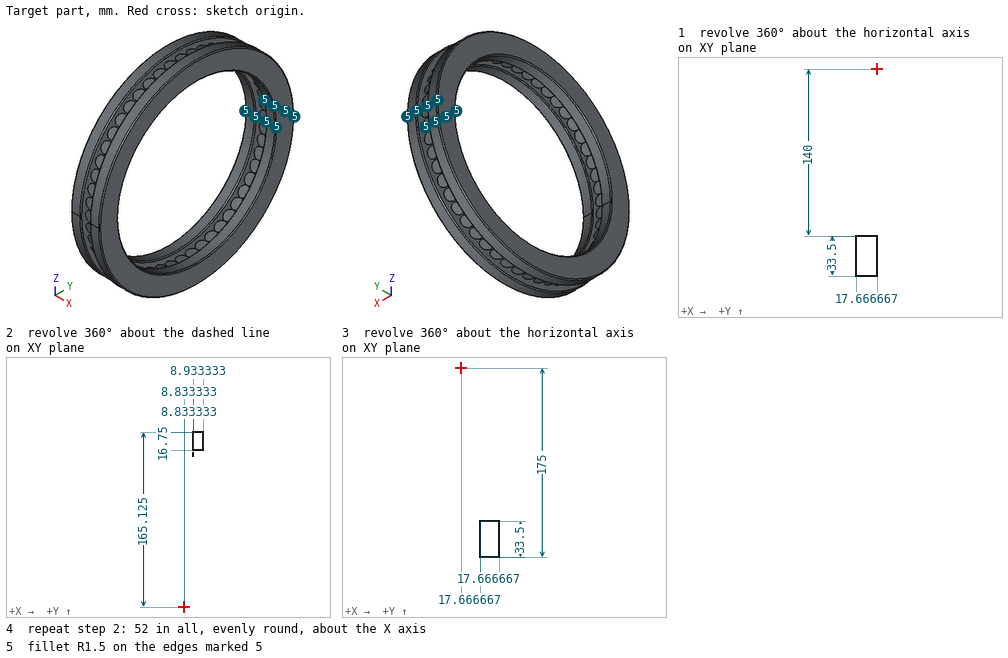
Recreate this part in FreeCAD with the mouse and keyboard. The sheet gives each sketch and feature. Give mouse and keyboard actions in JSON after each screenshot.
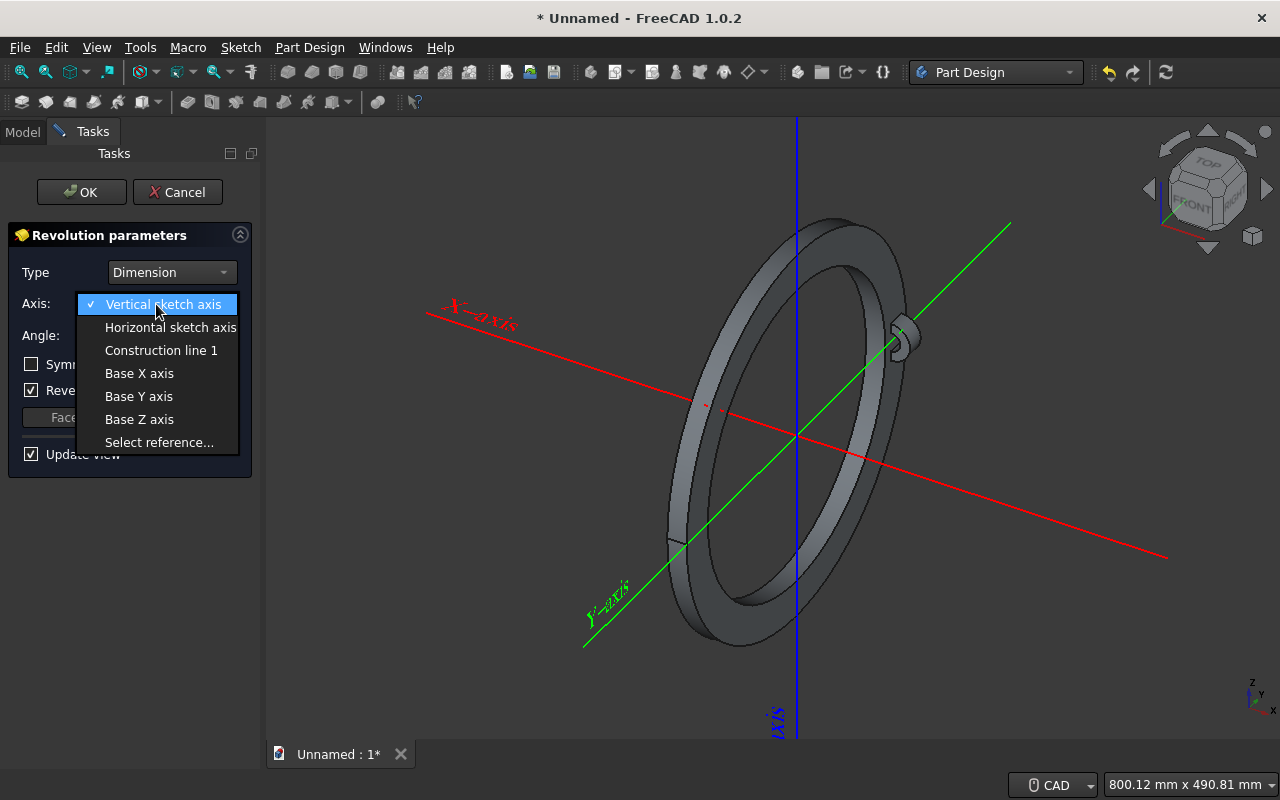
{"action": "left_click", "coordinate": [156, 350]}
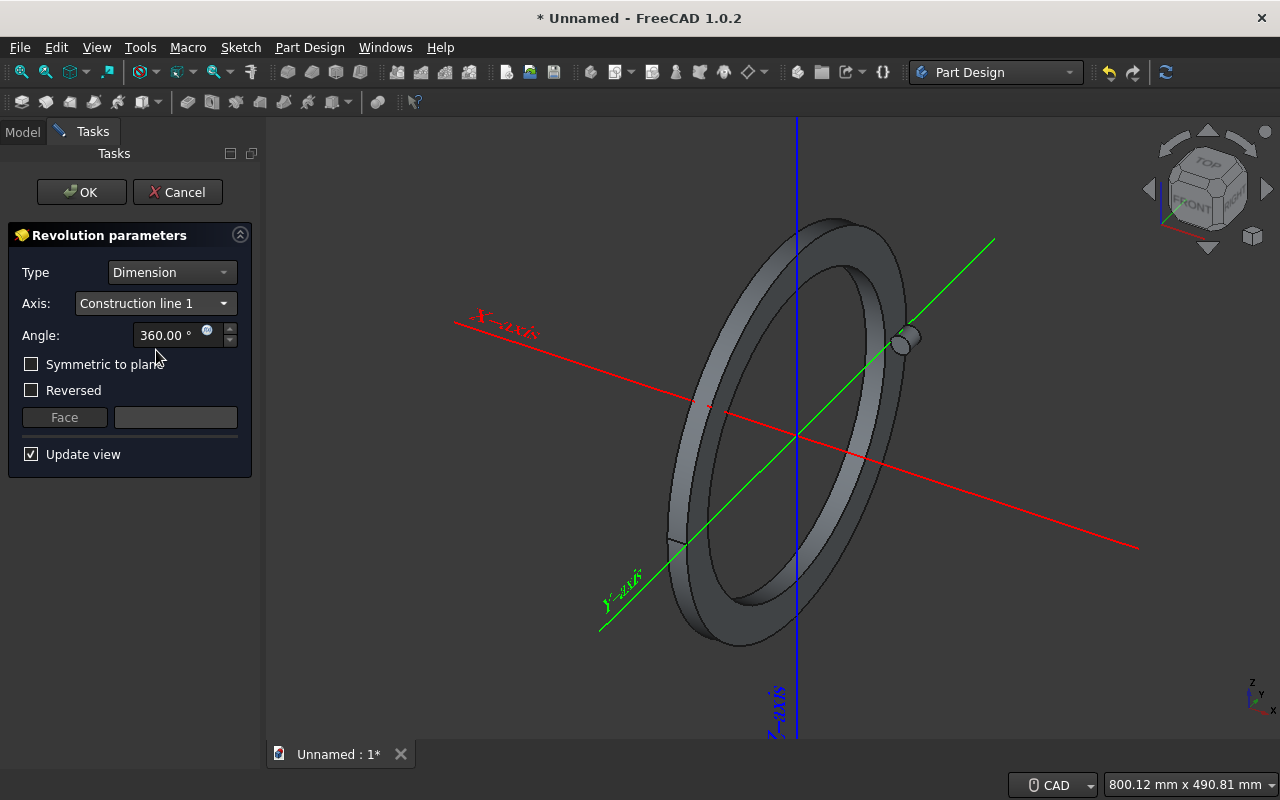
{"action": "left_click", "coordinate": [82, 192]}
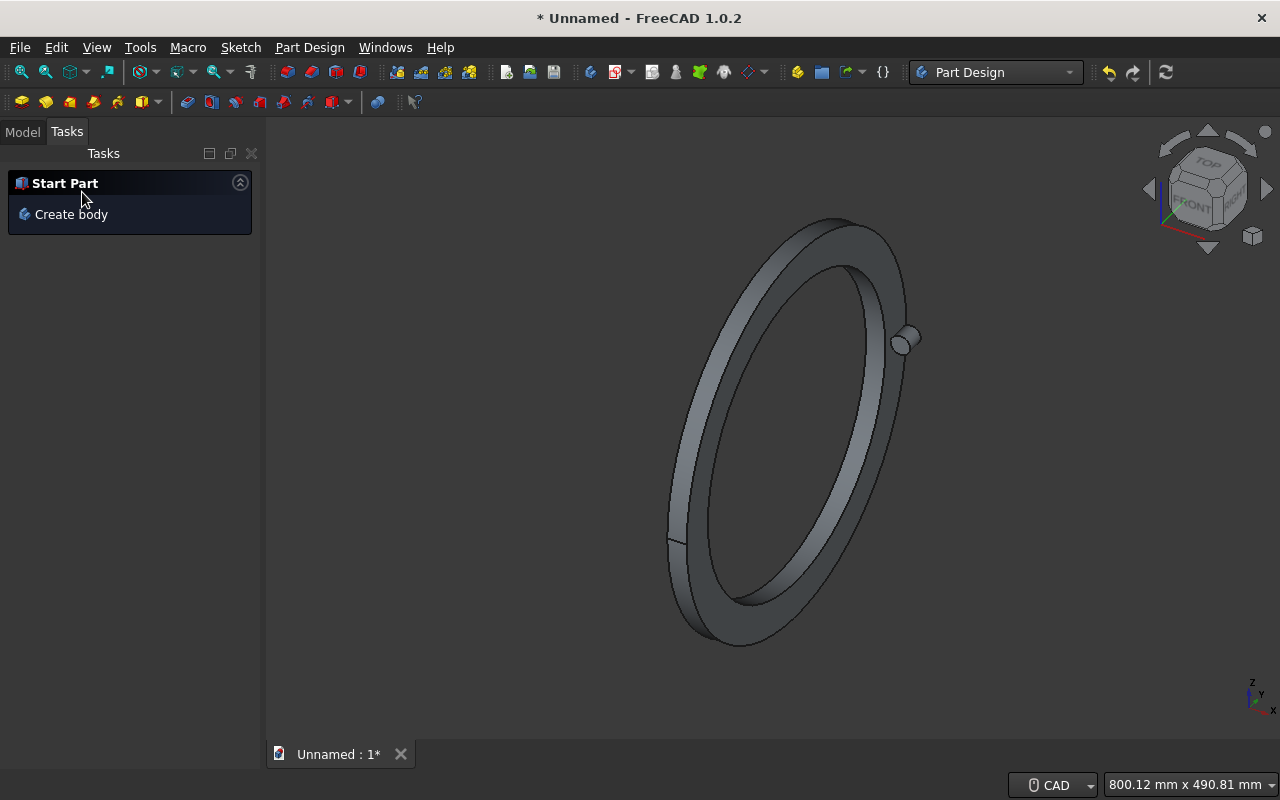
{"action": "left_click", "coordinate": [616, 72]}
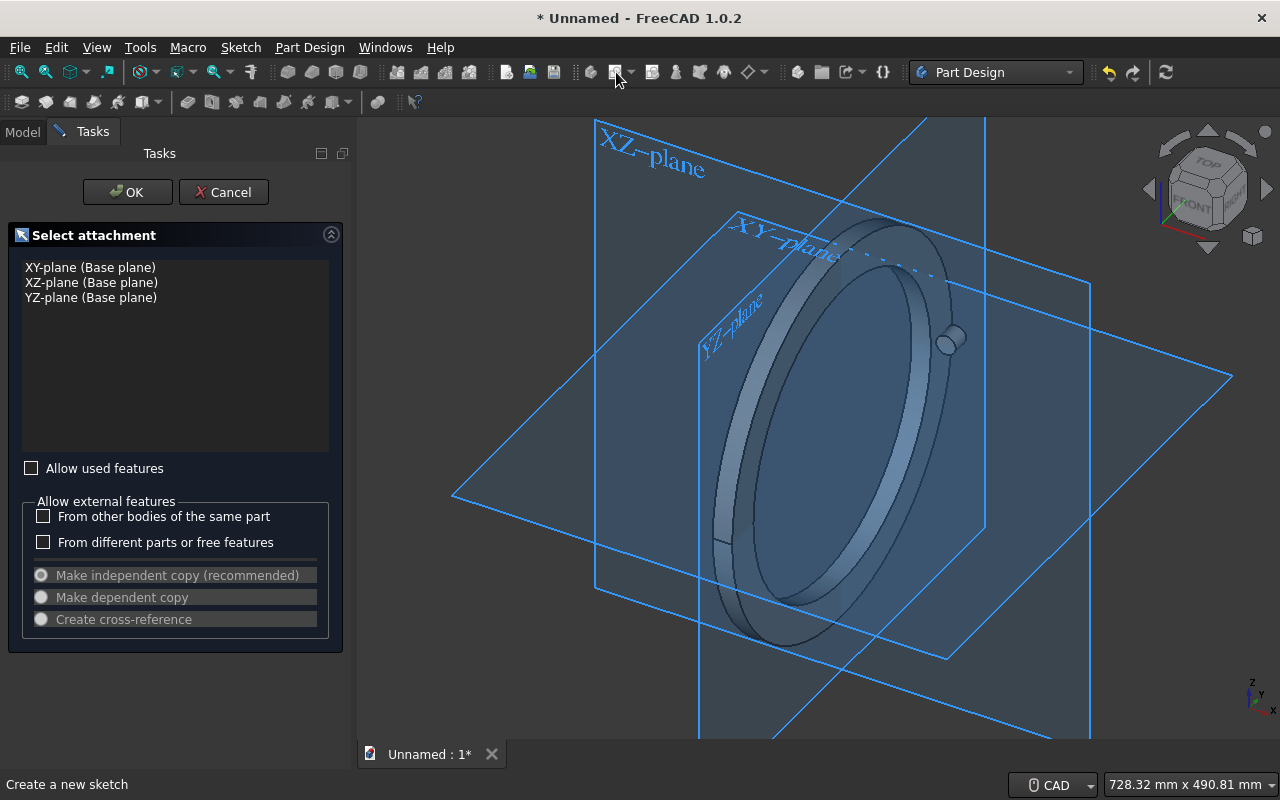
{"action": "left_click", "coordinate": [82, 268]}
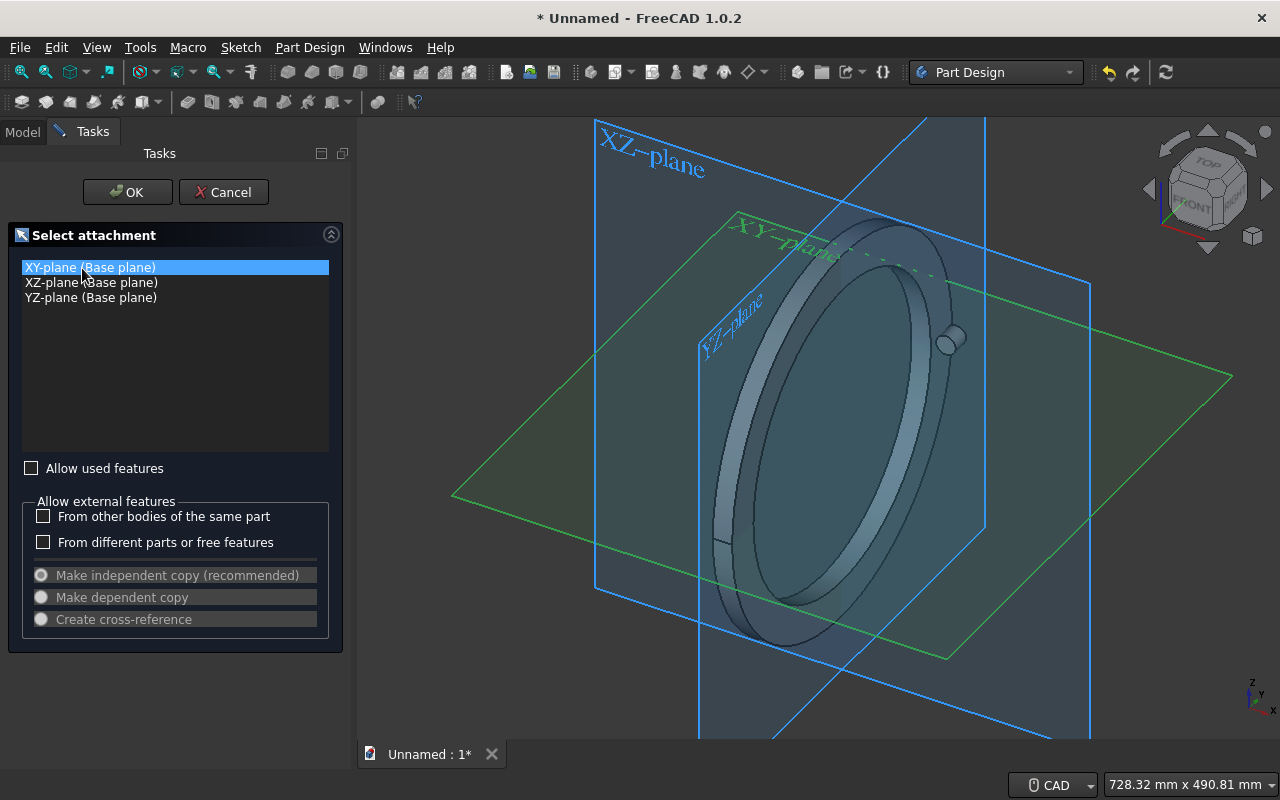
{"action": "left_click", "coordinate": [128, 192]}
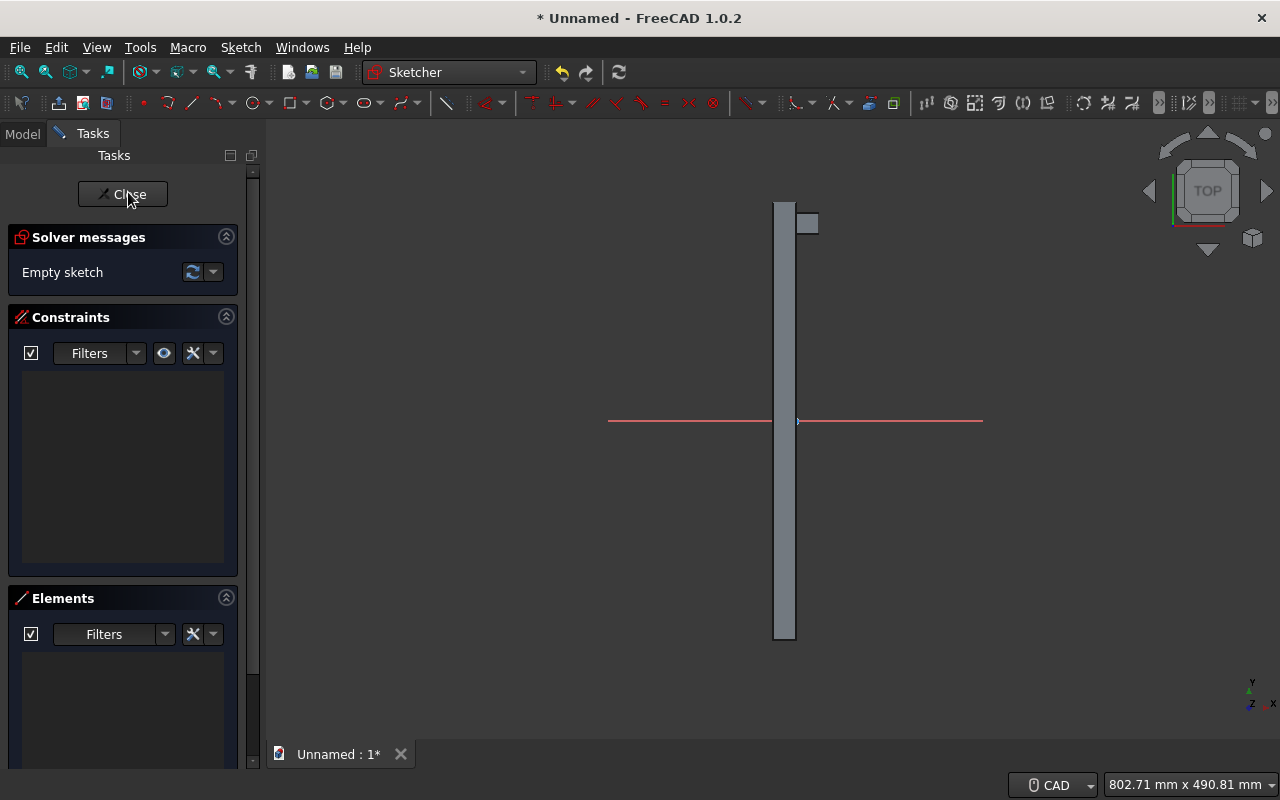
{"action": "left_click", "coordinate": [108, 104]}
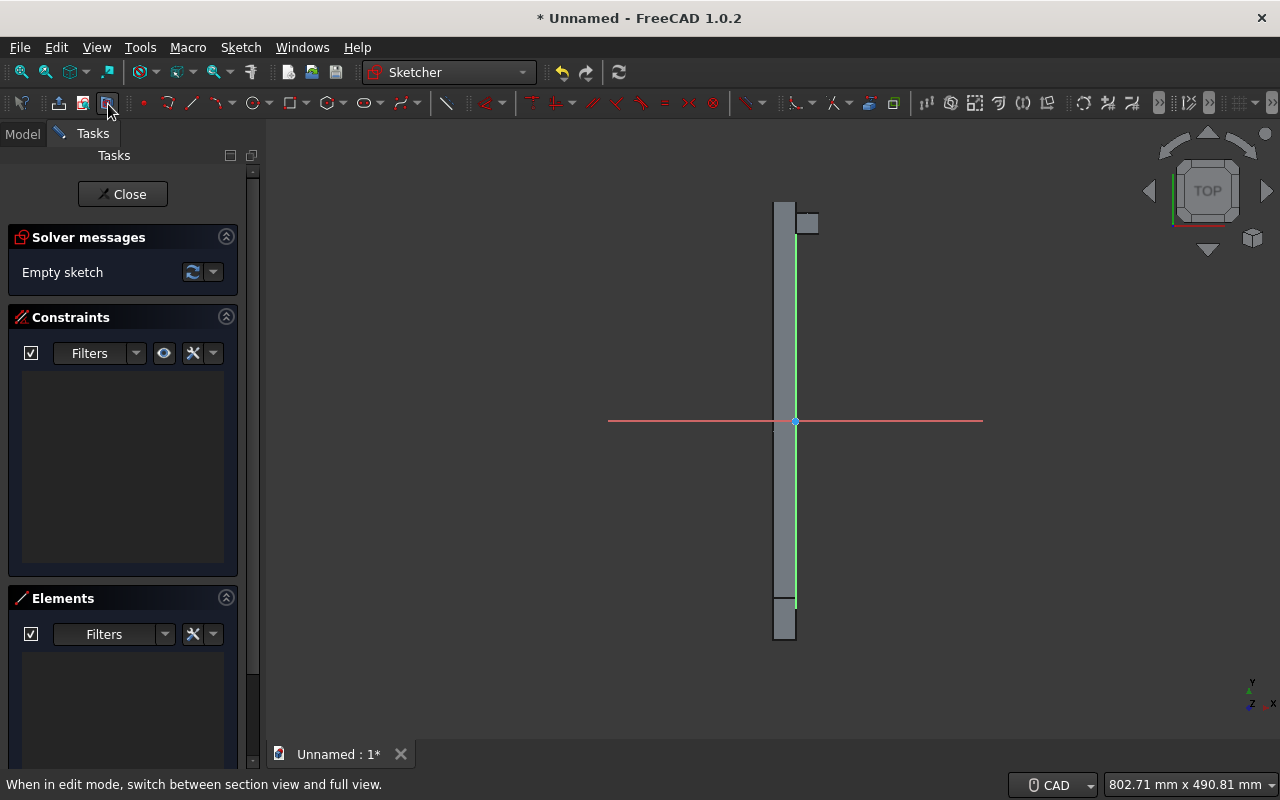
{"action": "scroll", "coordinate": [845, 645], "scroll_direction": "up", "scroll_amount": 11}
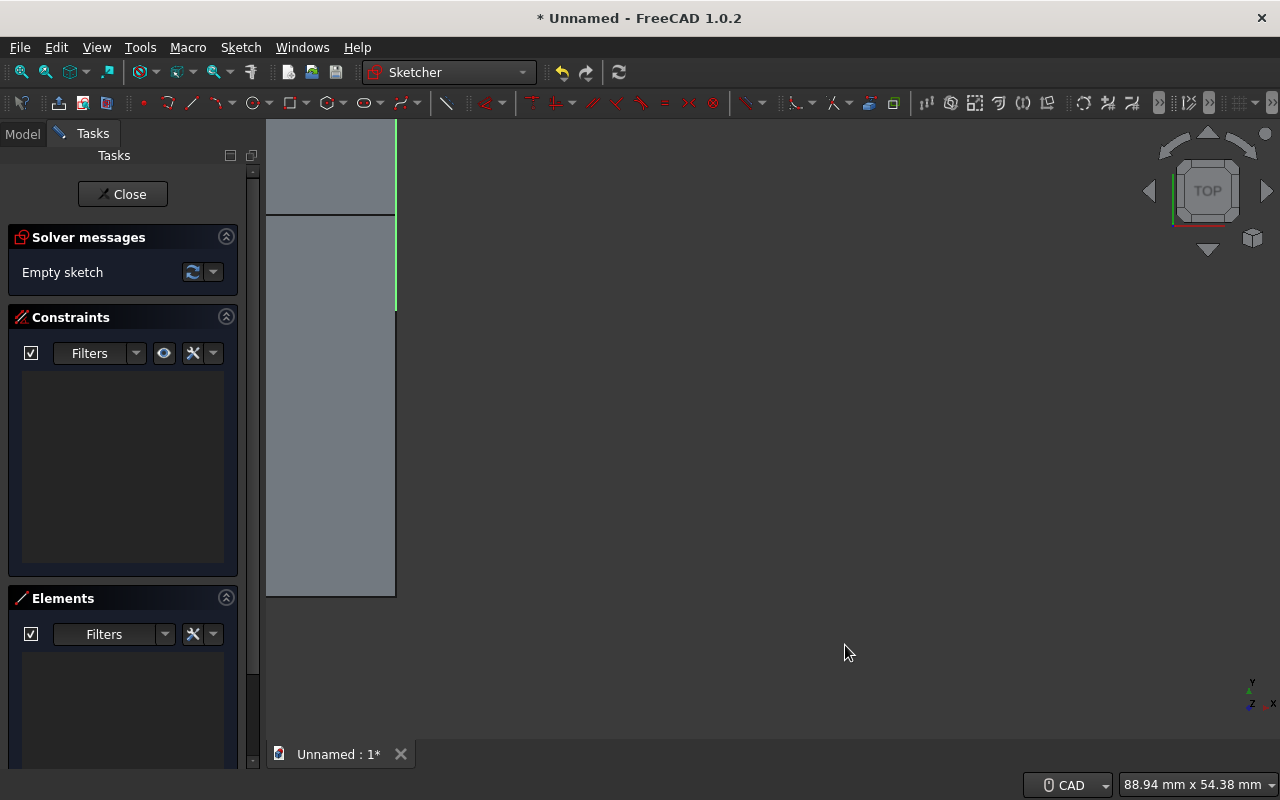
{"action": "left_click", "coordinate": [290, 104]}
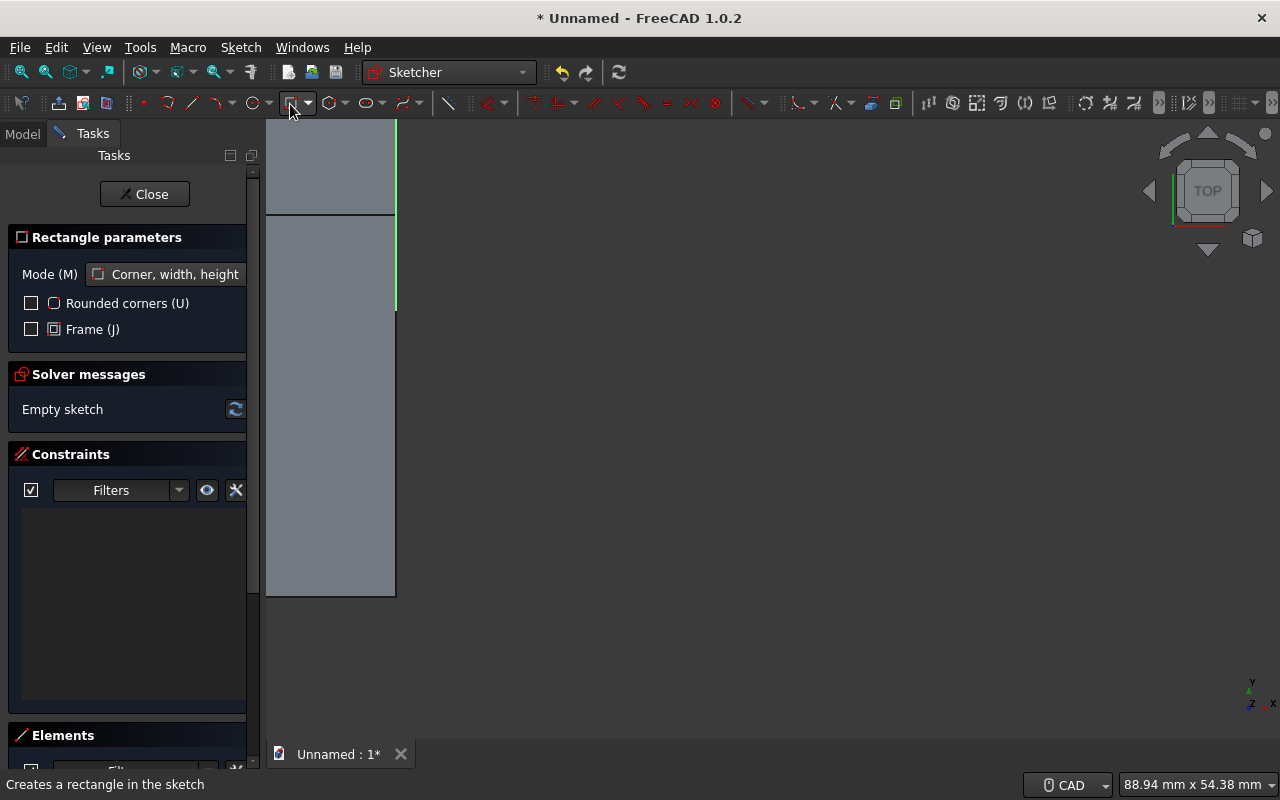
{"action": "left_click", "coordinate": [597, 232]}
{"action": "left_click", "coordinate": [799, 614]}
{"action": "key", "text": "Escape"}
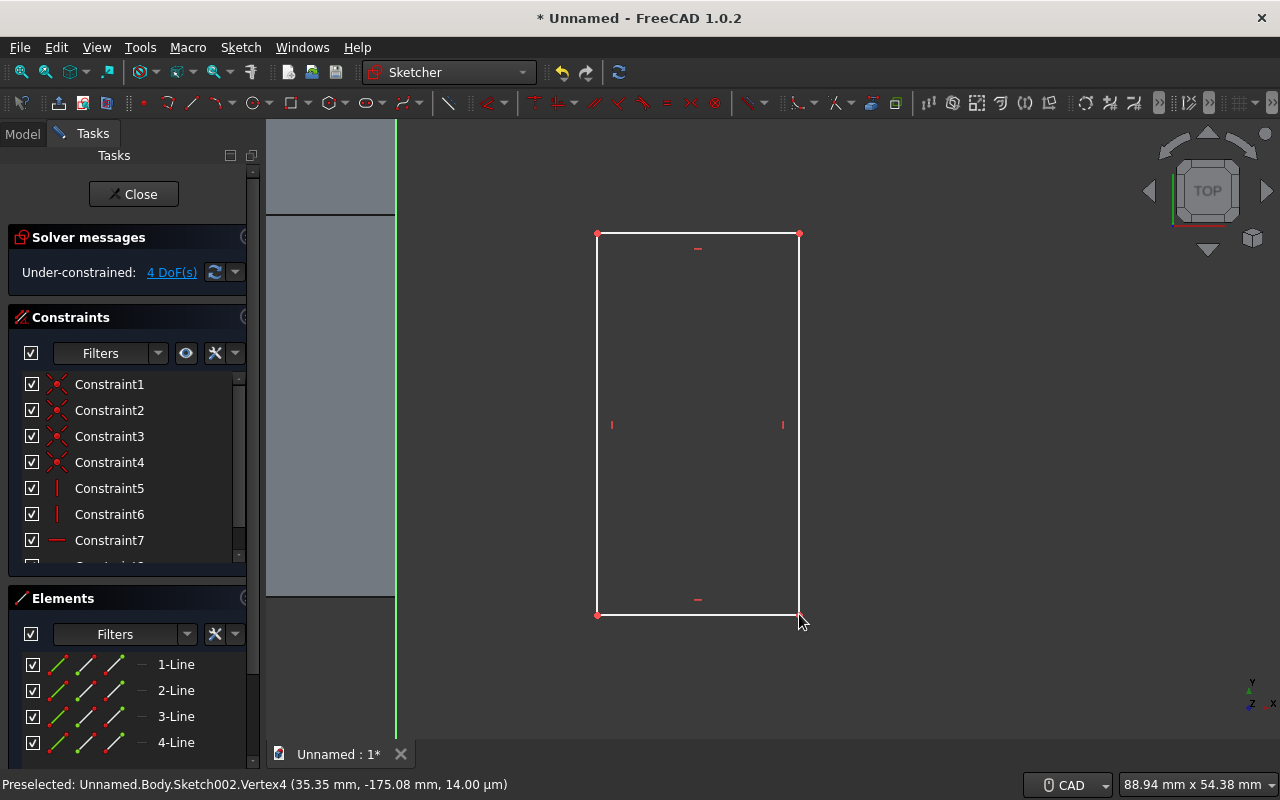
{"action": "left_click", "coordinate": [488, 104]}